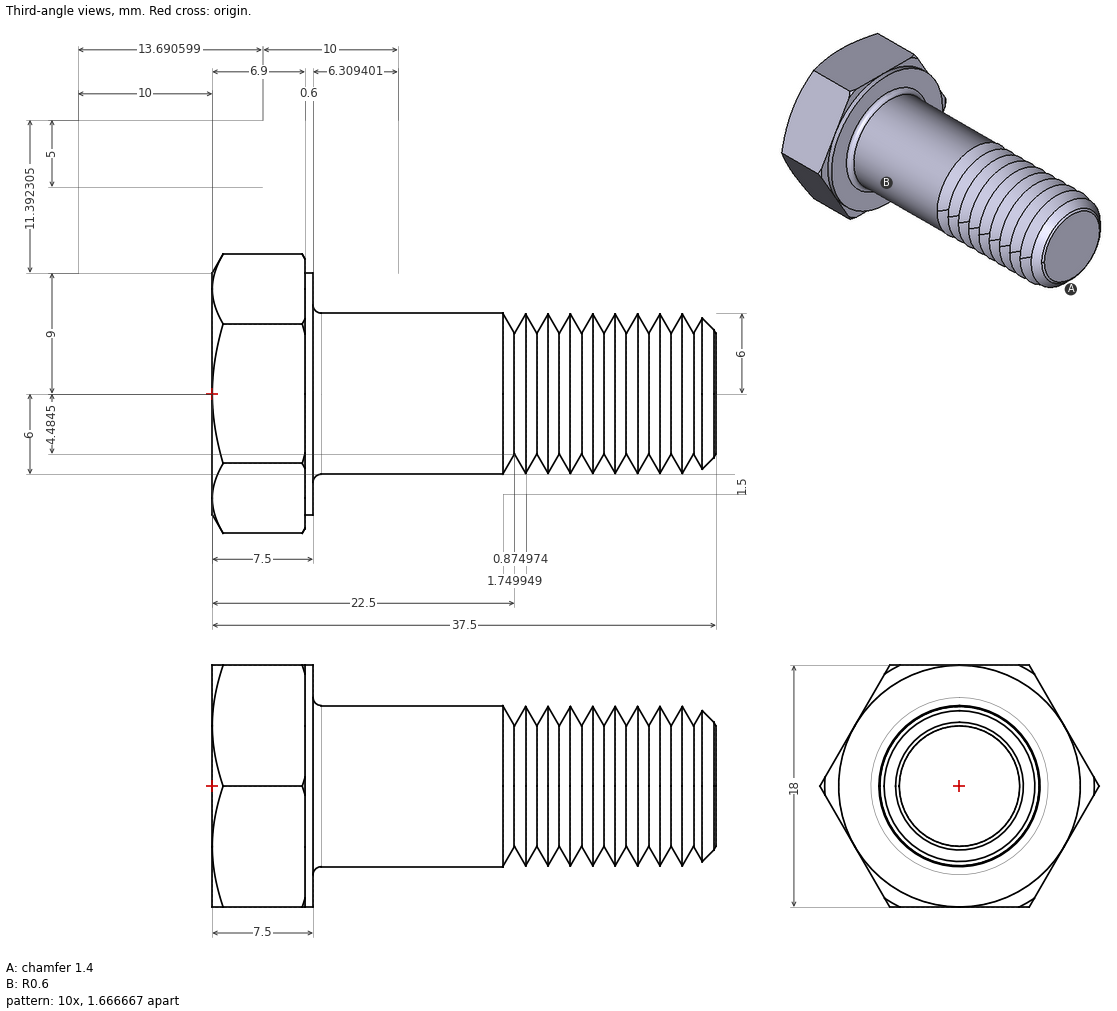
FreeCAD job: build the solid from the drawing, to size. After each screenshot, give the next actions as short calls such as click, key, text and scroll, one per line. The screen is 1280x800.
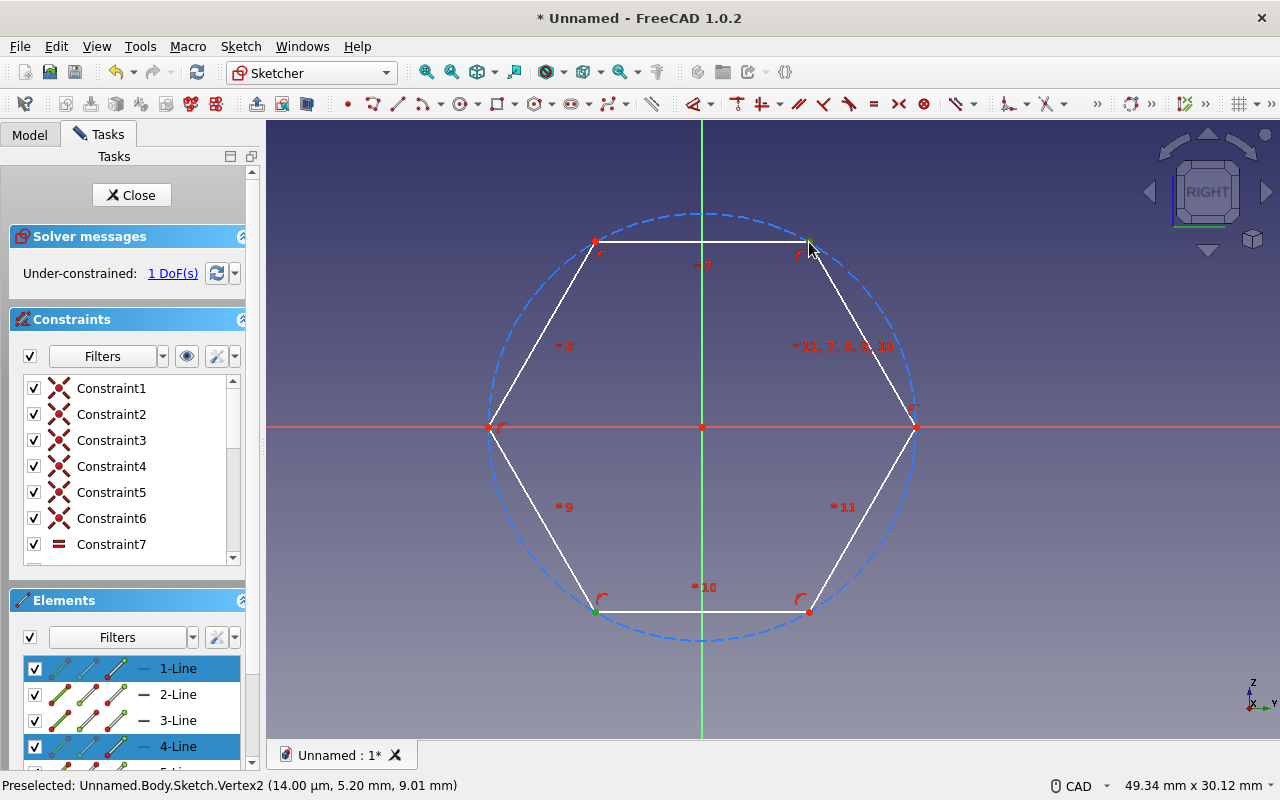
key(i)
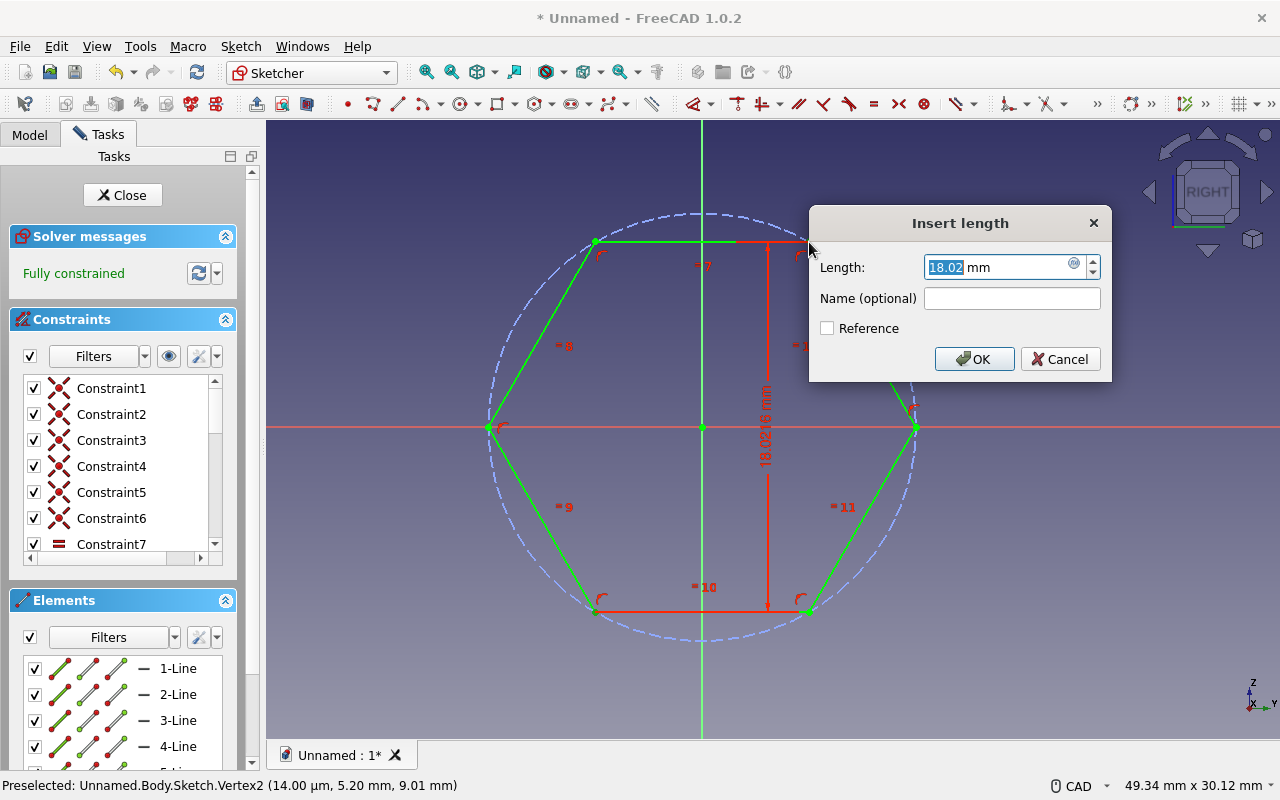
text(18)
key(Return)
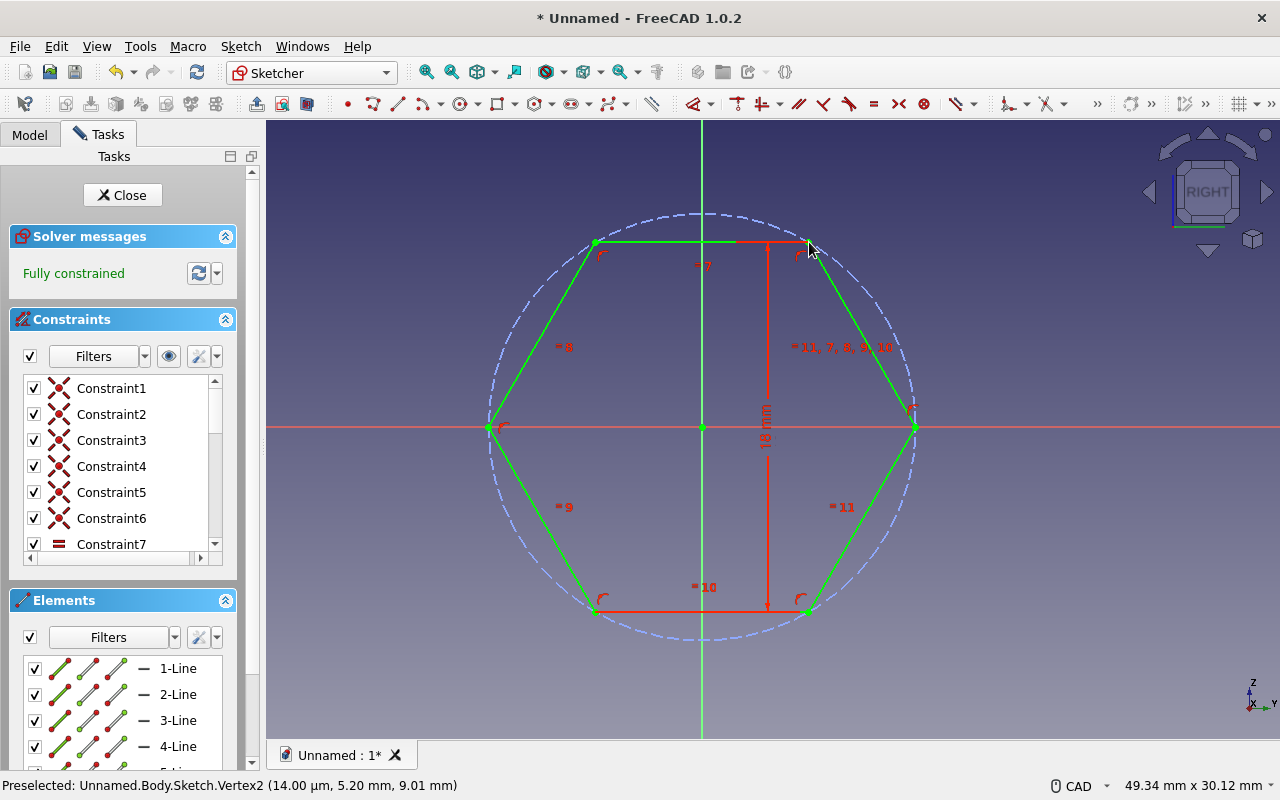
click(123, 195)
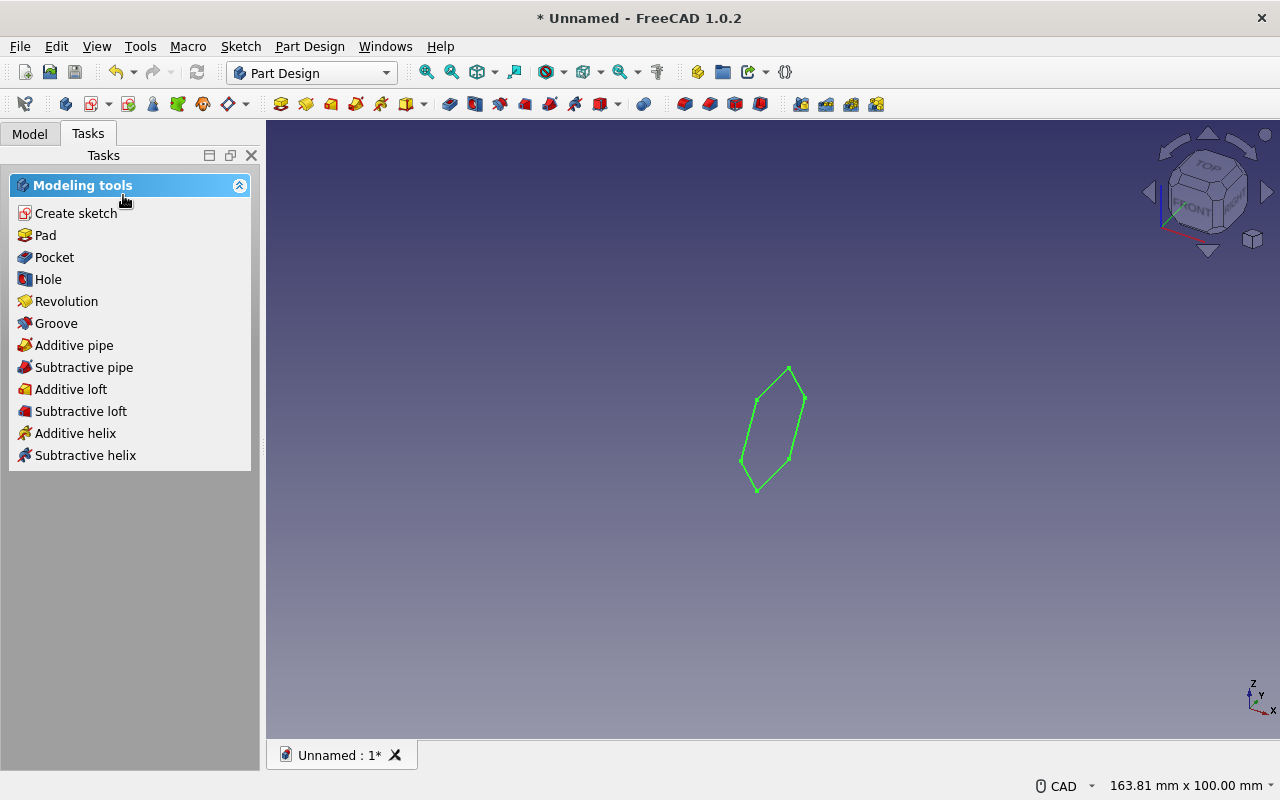
click(281, 104)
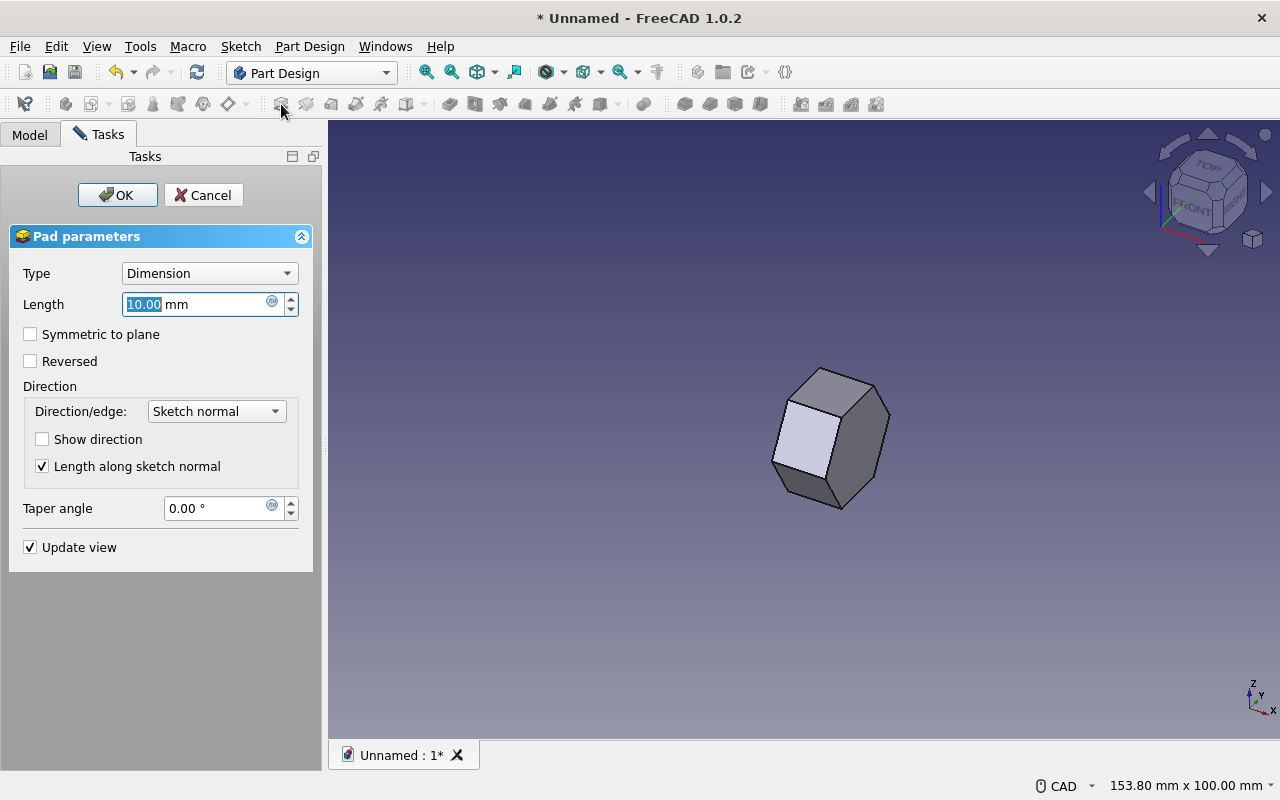
text(7.5)
key(Tab)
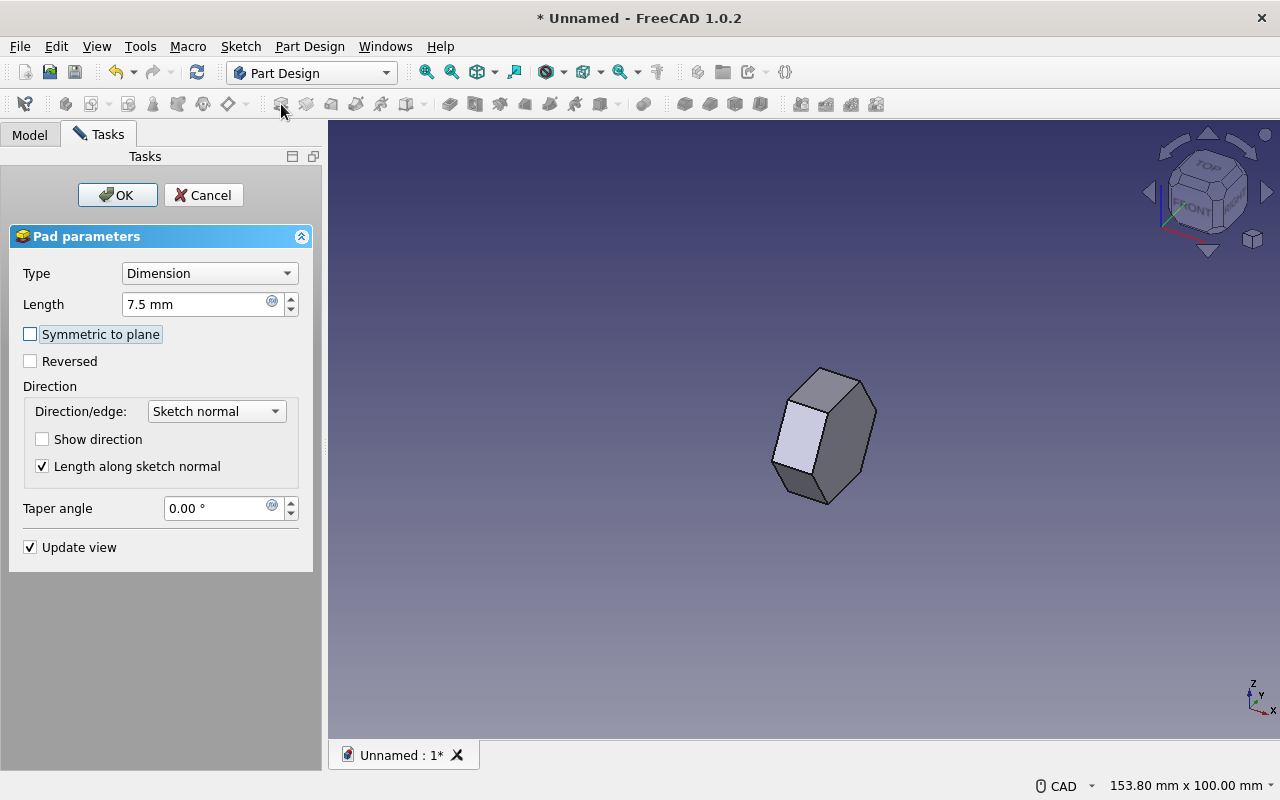
click(118, 195)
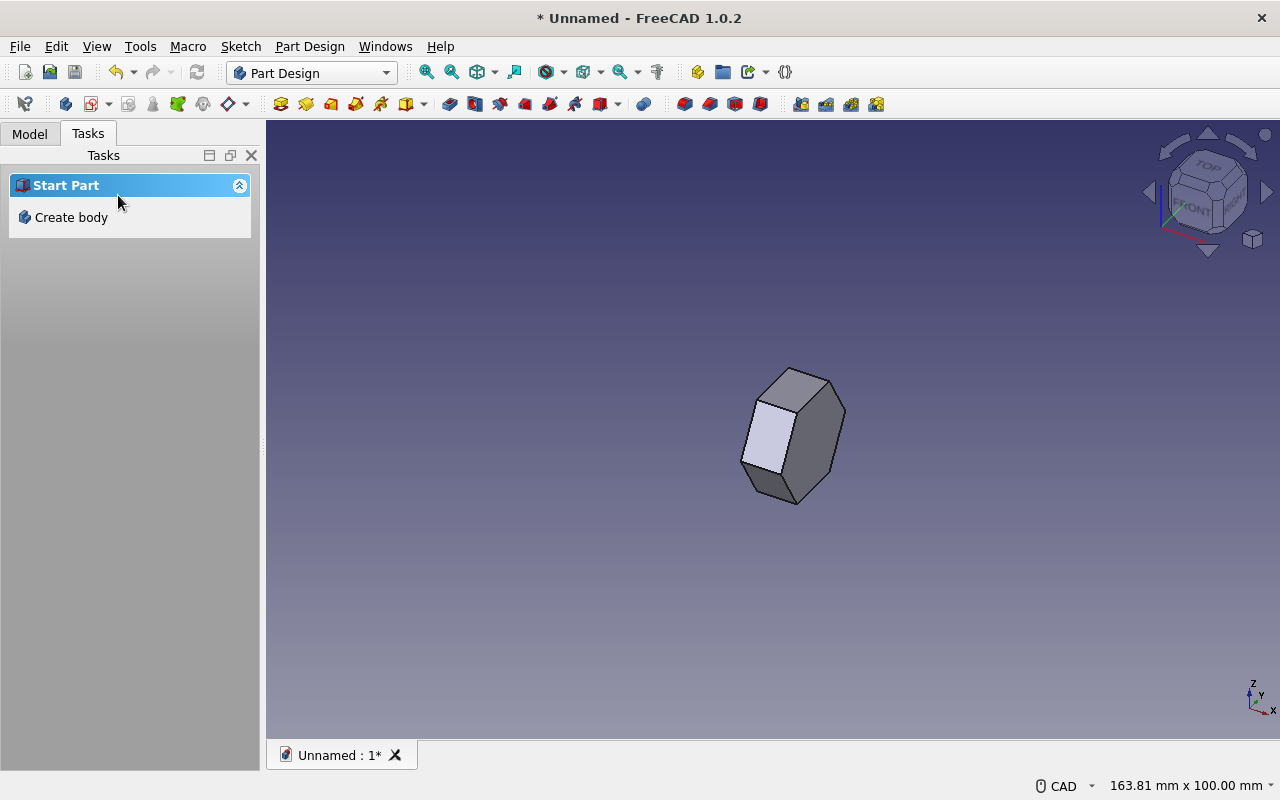
click(427, 72)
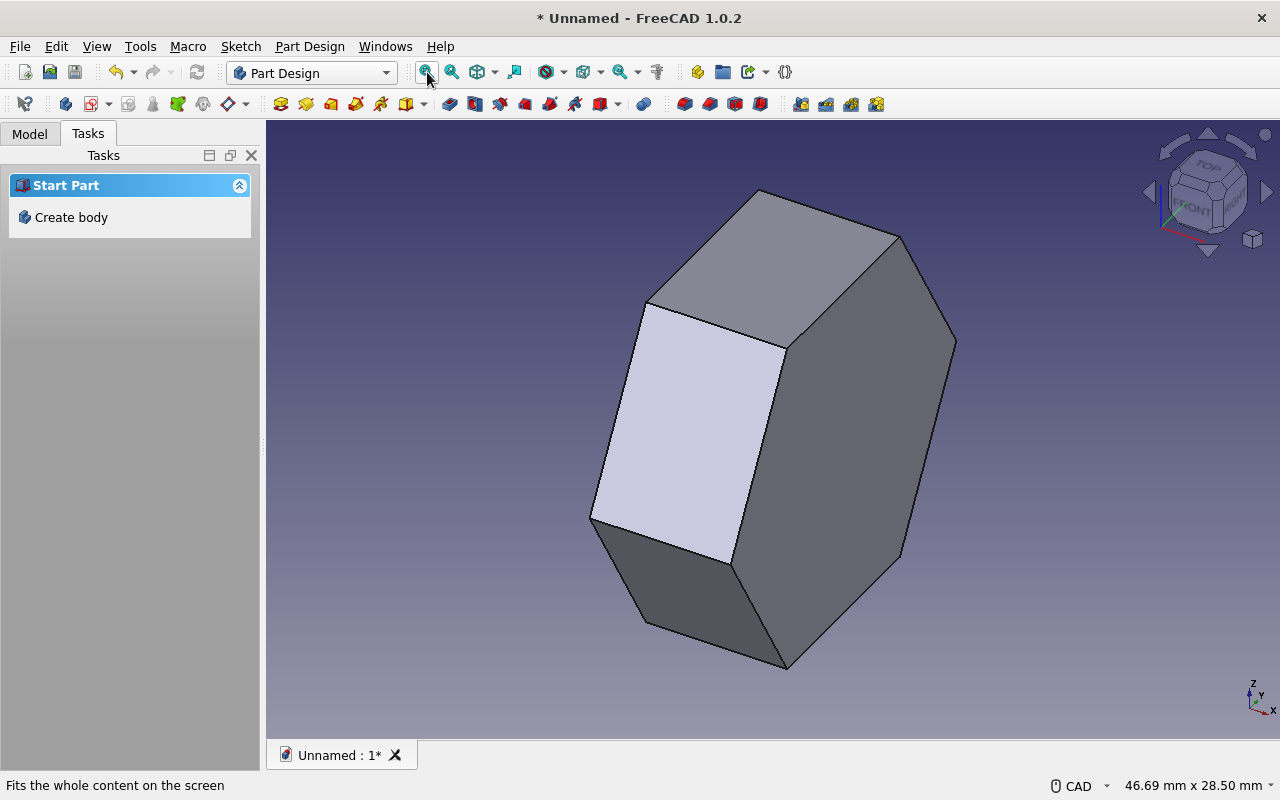
click(90, 104)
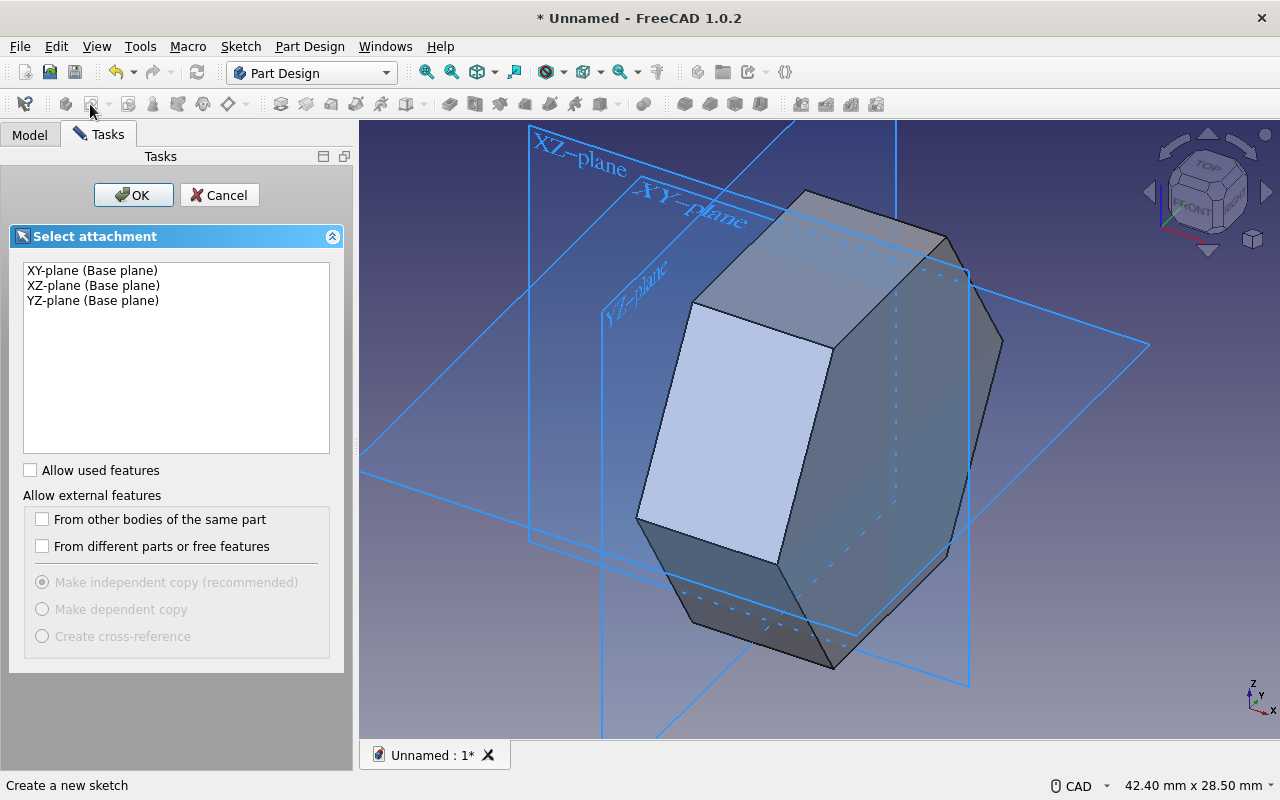
click(84, 270)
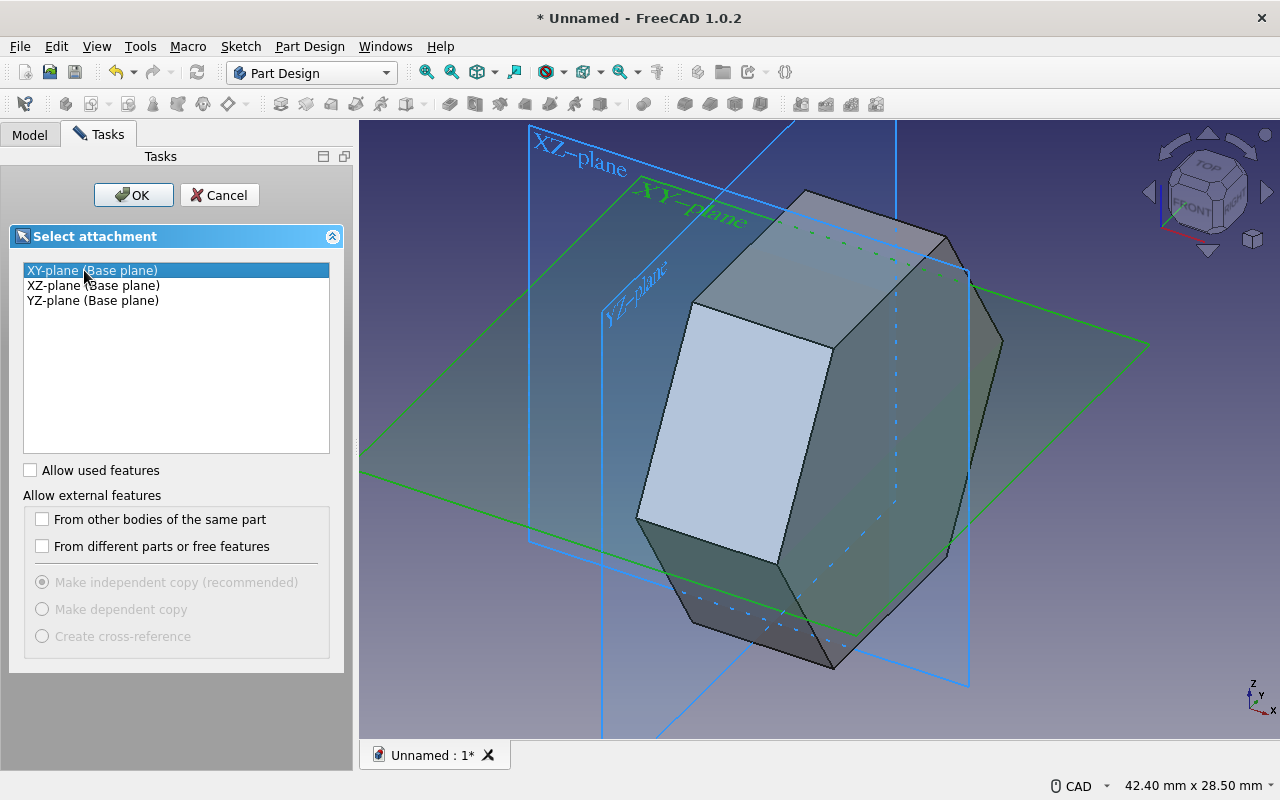
click(134, 195)